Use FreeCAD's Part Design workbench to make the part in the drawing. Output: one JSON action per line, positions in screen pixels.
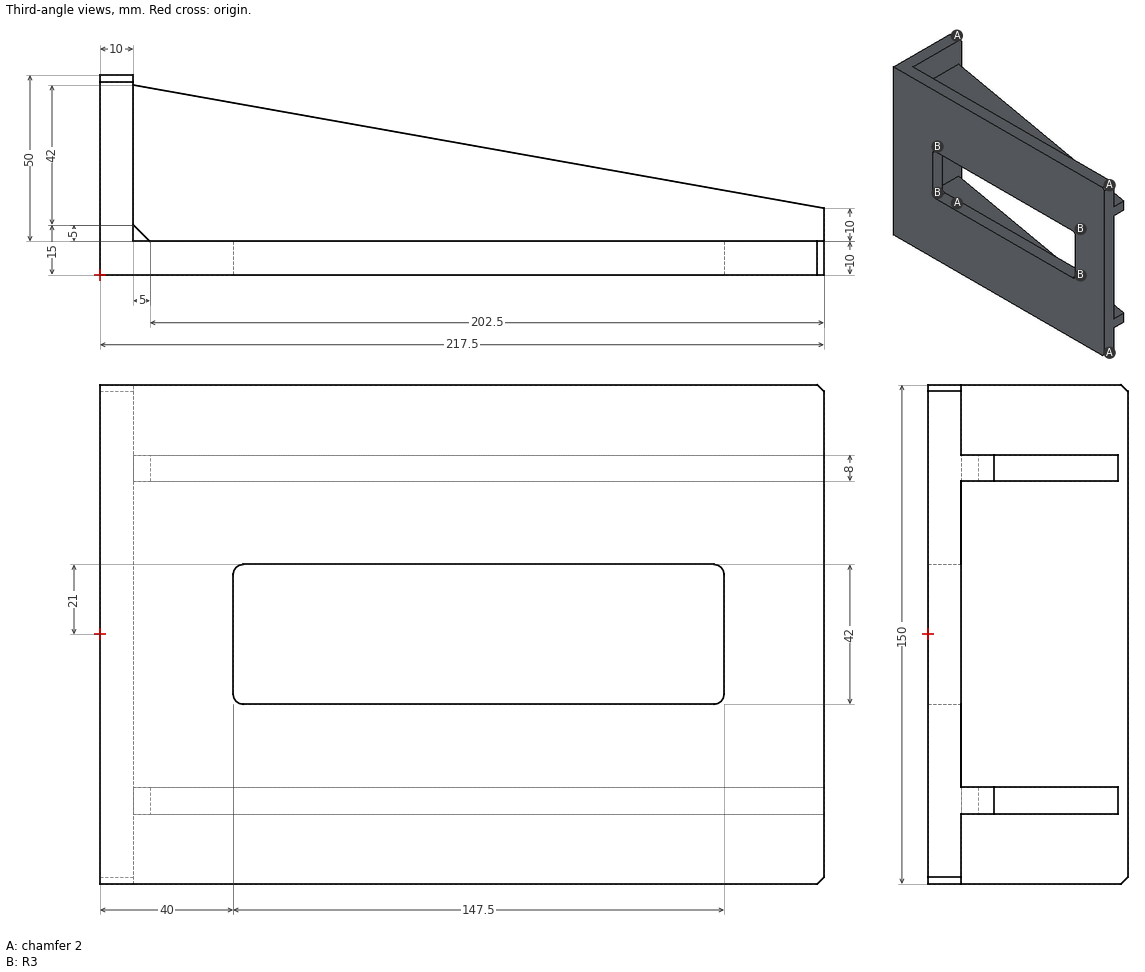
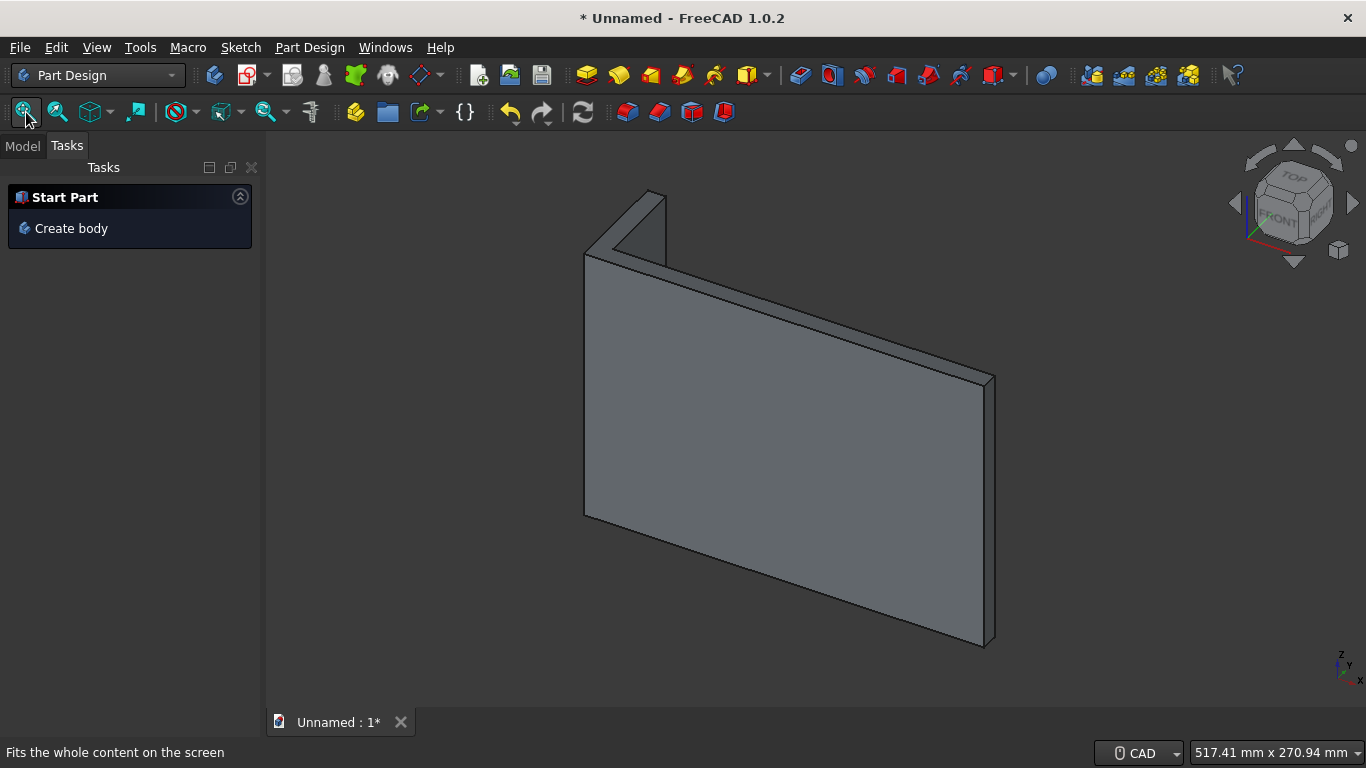
{"action": "left_click", "coordinate": [23, 145]}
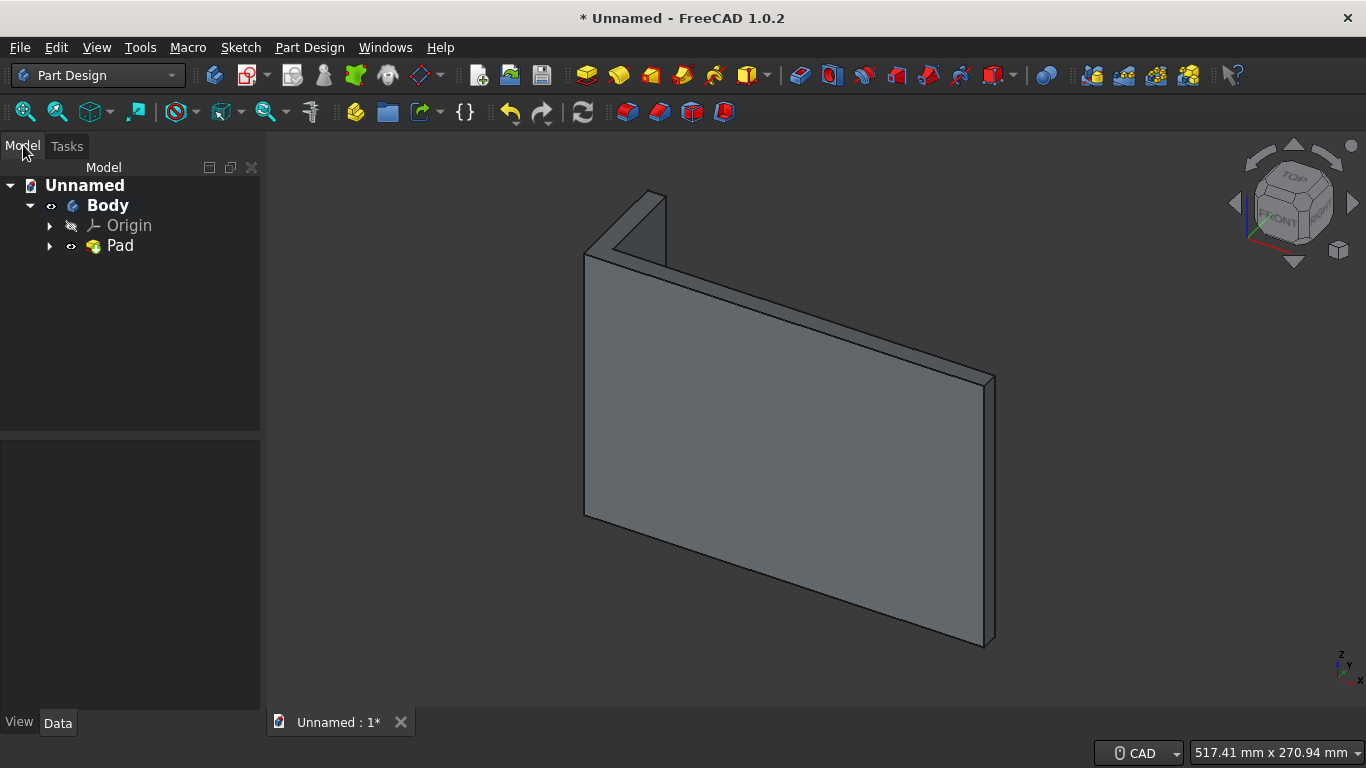
{"action": "left_click", "coordinate": [50, 226]}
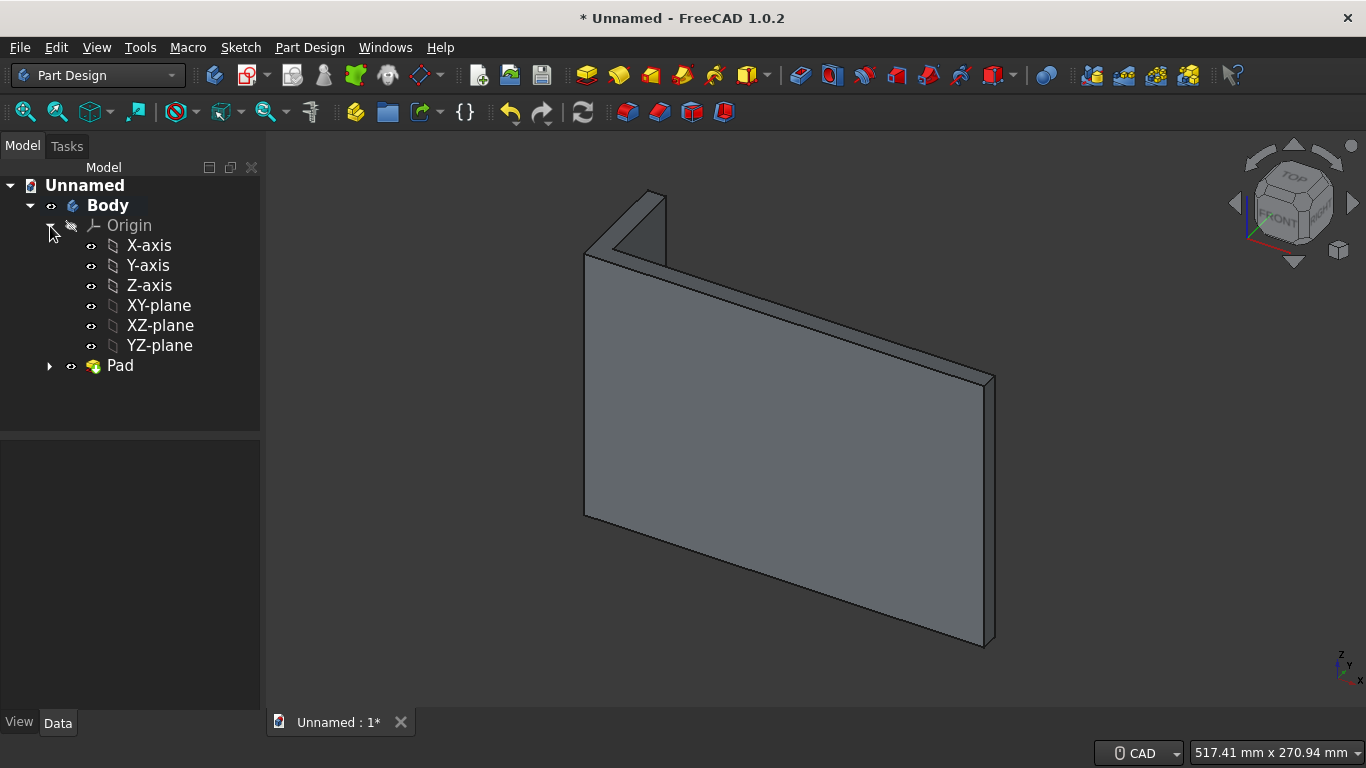
{"action": "left_click", "coordinate": [136, 306]}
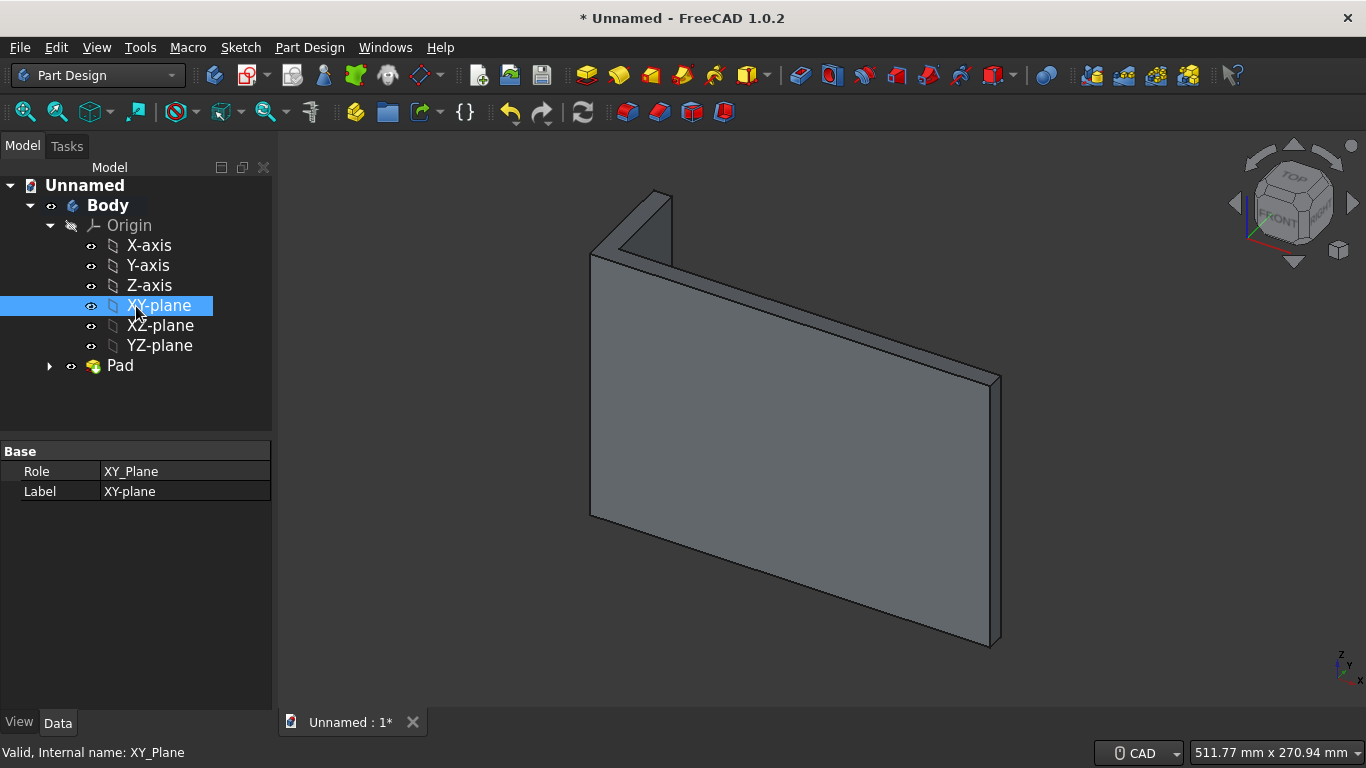
{"action": "left_click", "coordinate": [420, 76]}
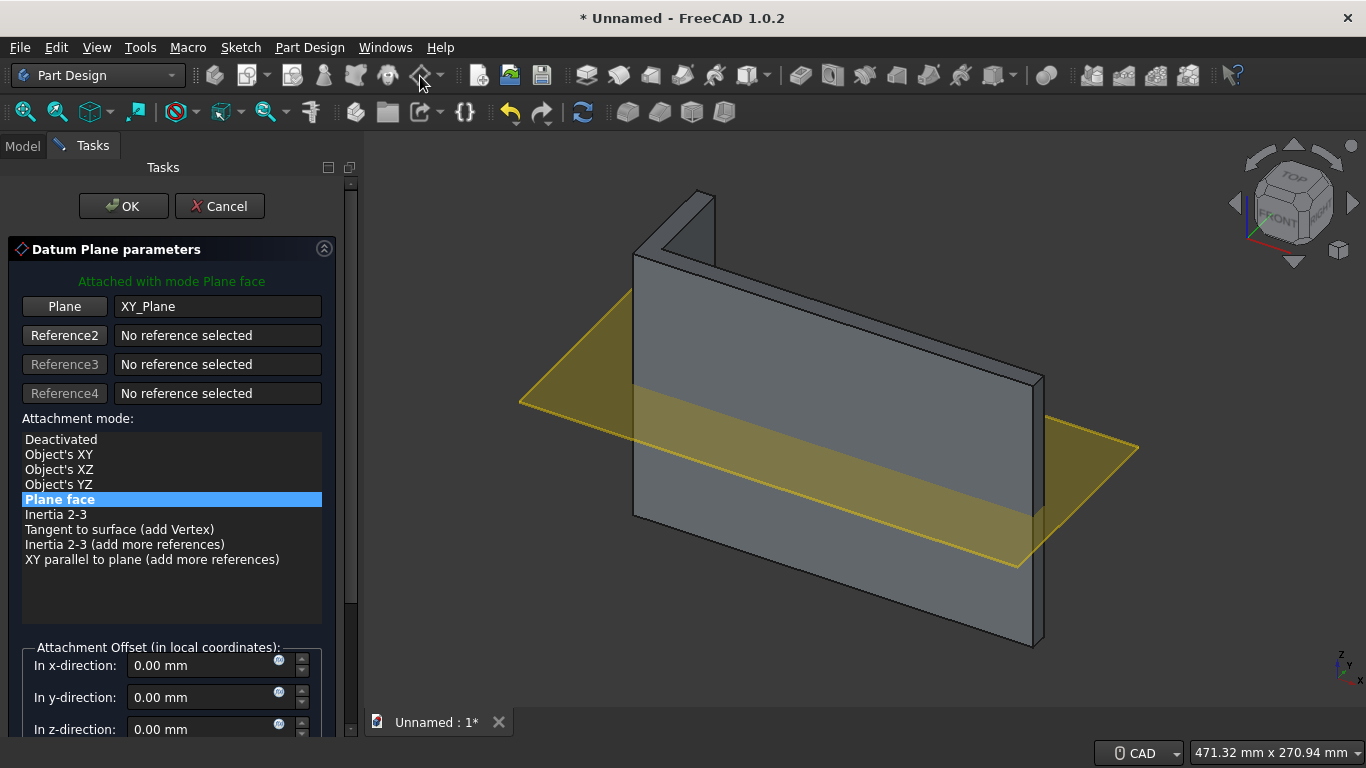
{"action": "scroll", "coordinate": [351, 456], "scroll_direction": "down", "scroll_amount": 2}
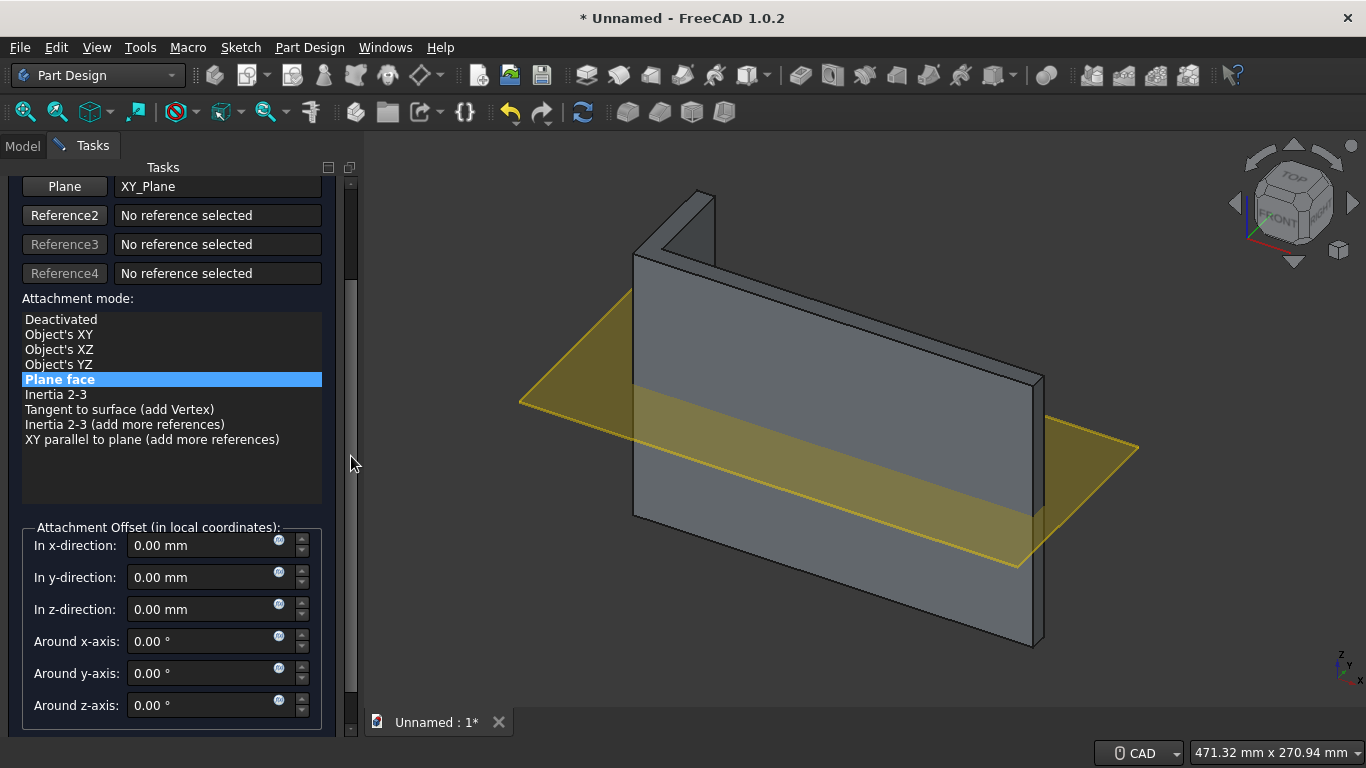
{"action": "triple_click", "coordinate": [210, 609]}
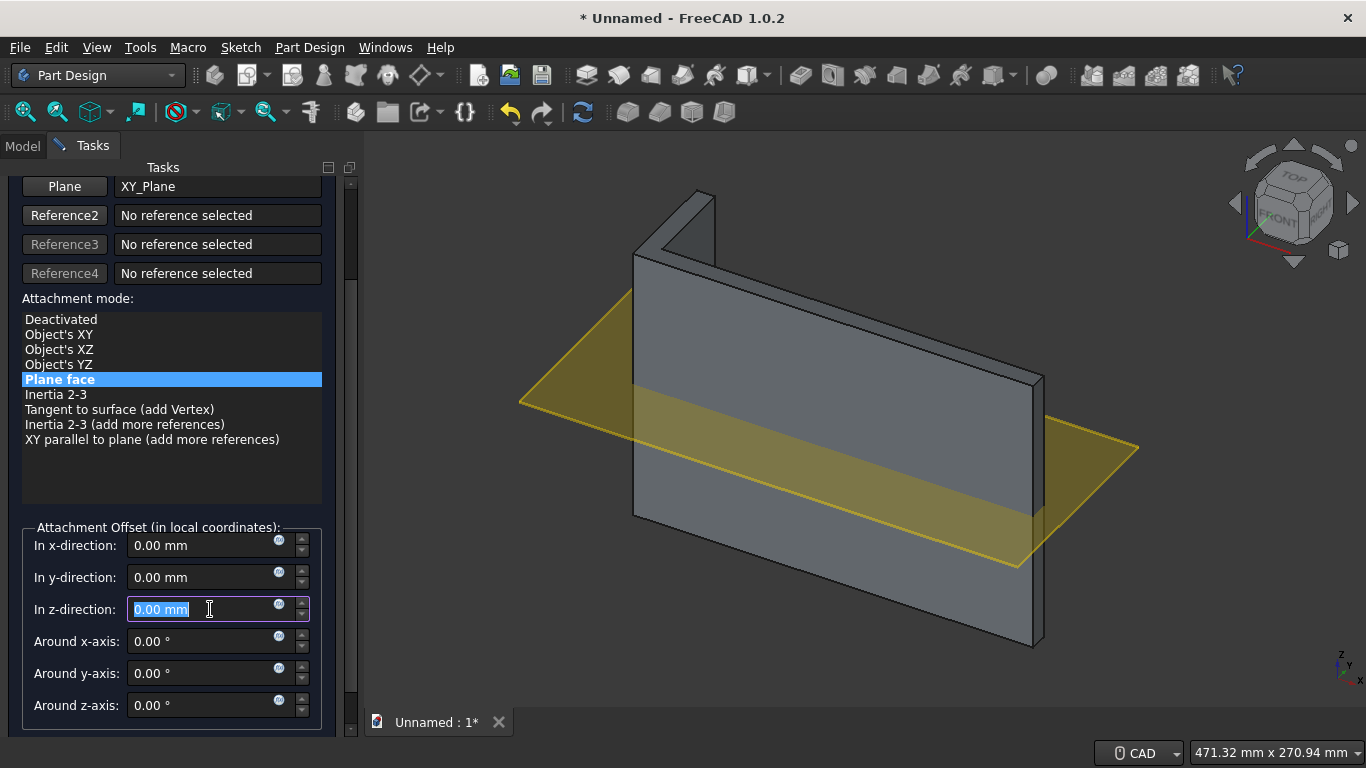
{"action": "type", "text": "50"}
{"action": "key", "text": "Tab"}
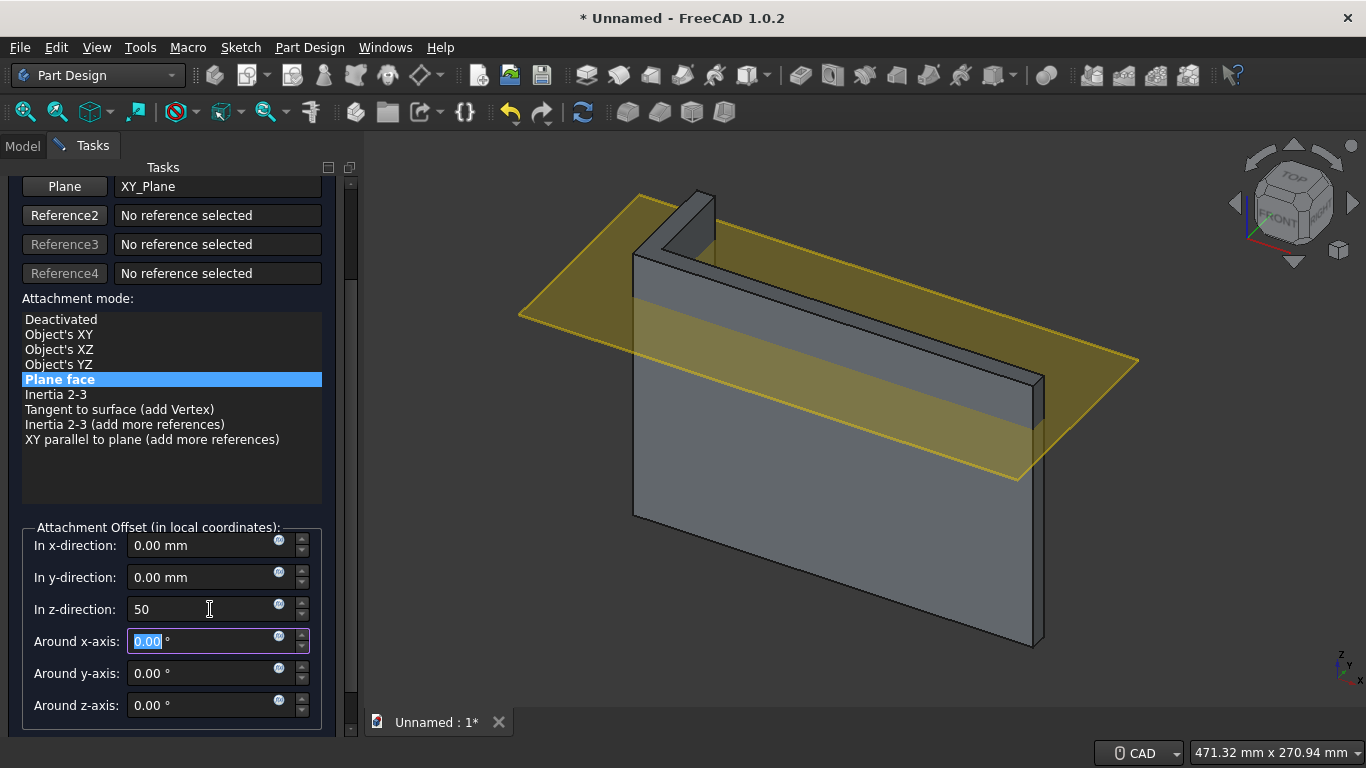
{"action": "scroll", "coordinate": [351, 456], "scroll_direction": "up", "scroll_amount": 3}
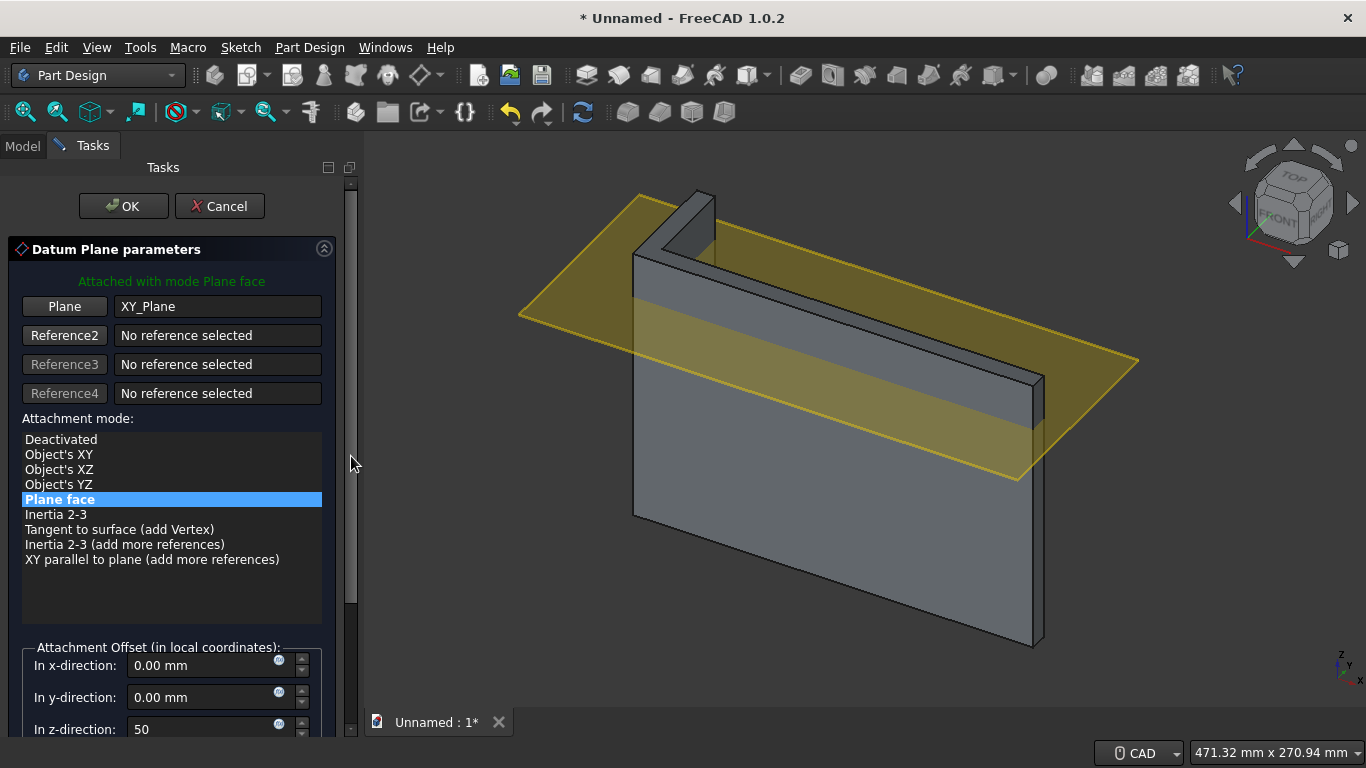
{"action": "left_click", "coordinate": [124, 206]}